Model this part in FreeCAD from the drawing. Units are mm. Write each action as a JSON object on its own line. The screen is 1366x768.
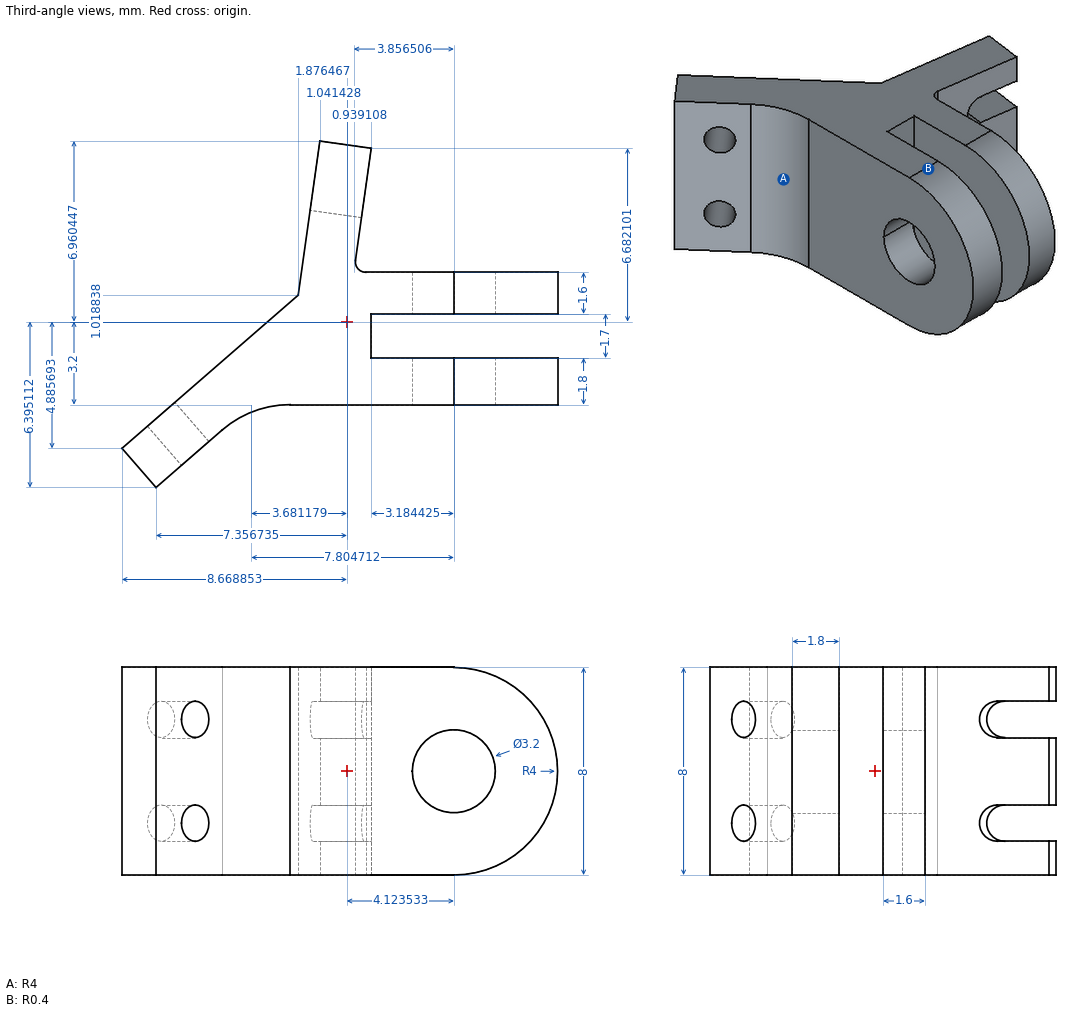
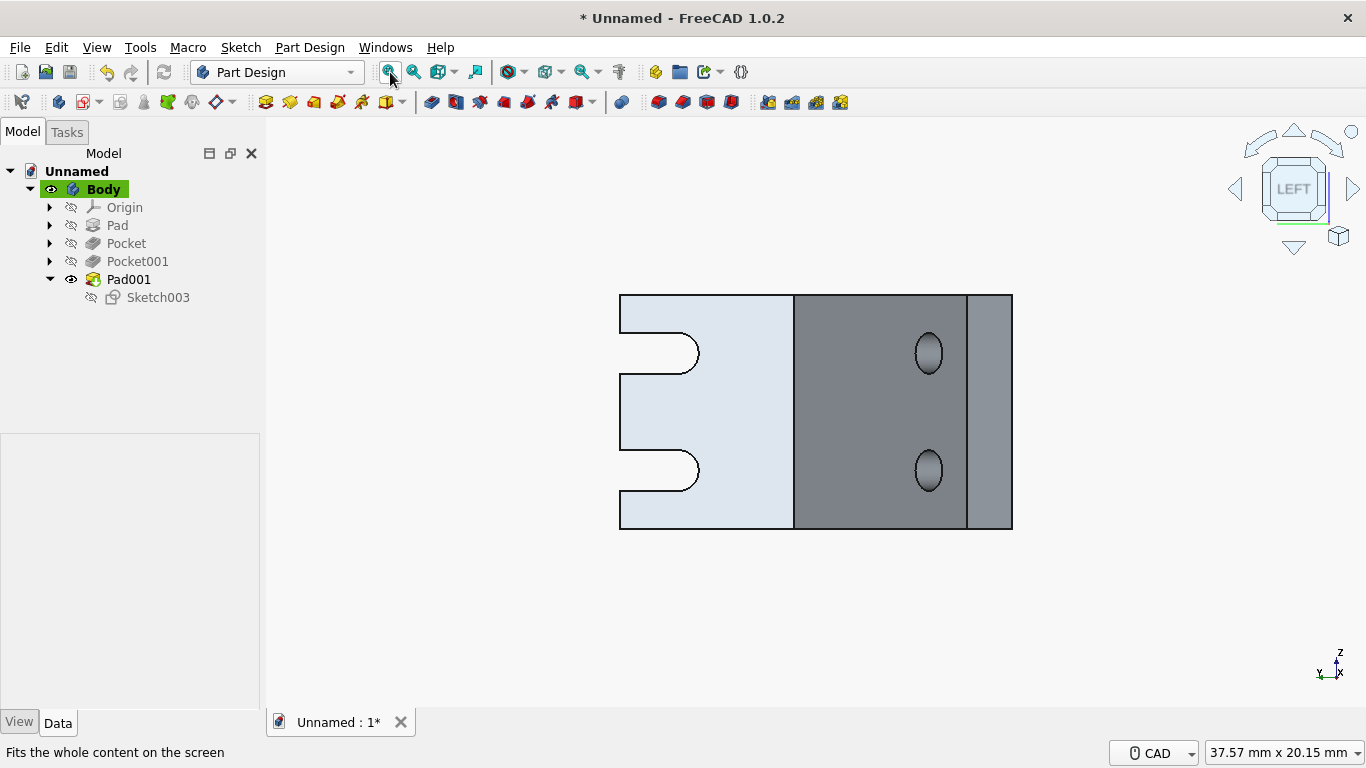
{"action": "key", "text": "v 3"}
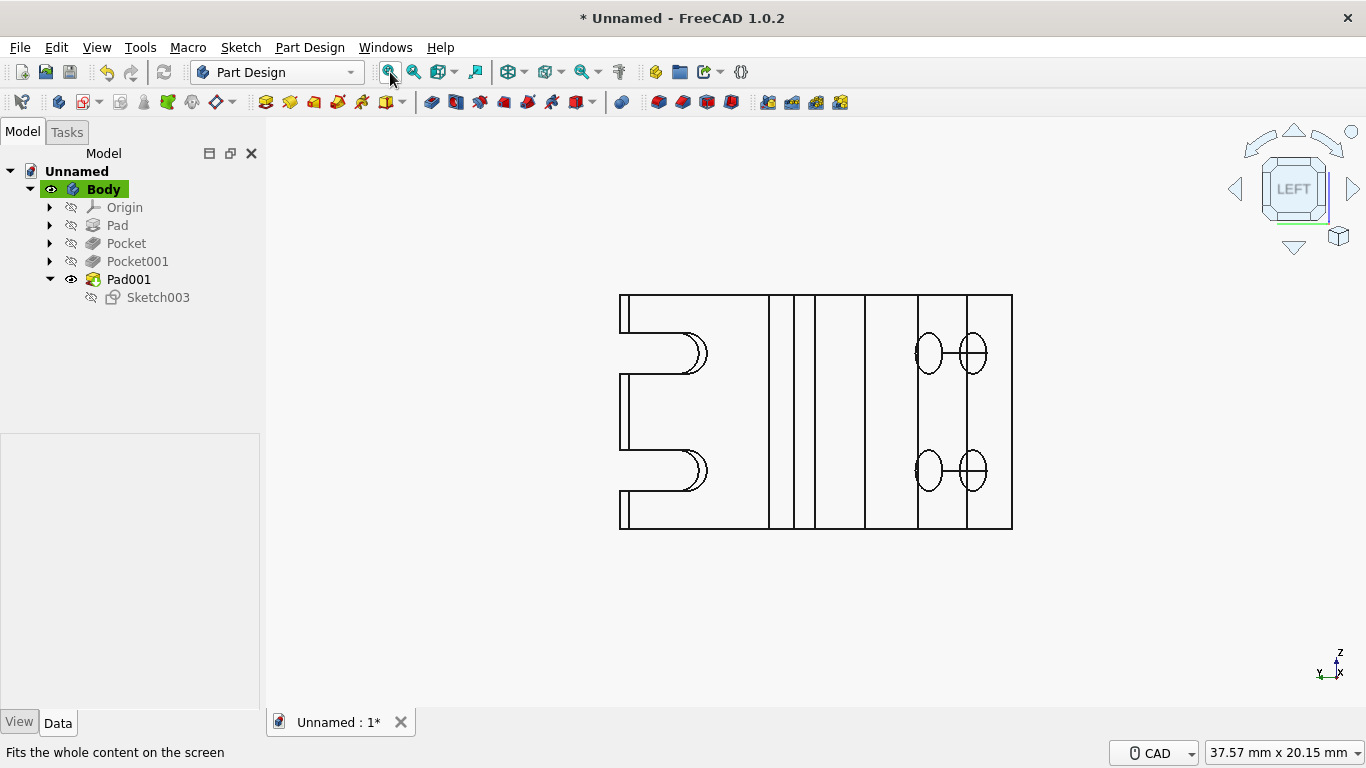
{"action": "key", "text": "0"}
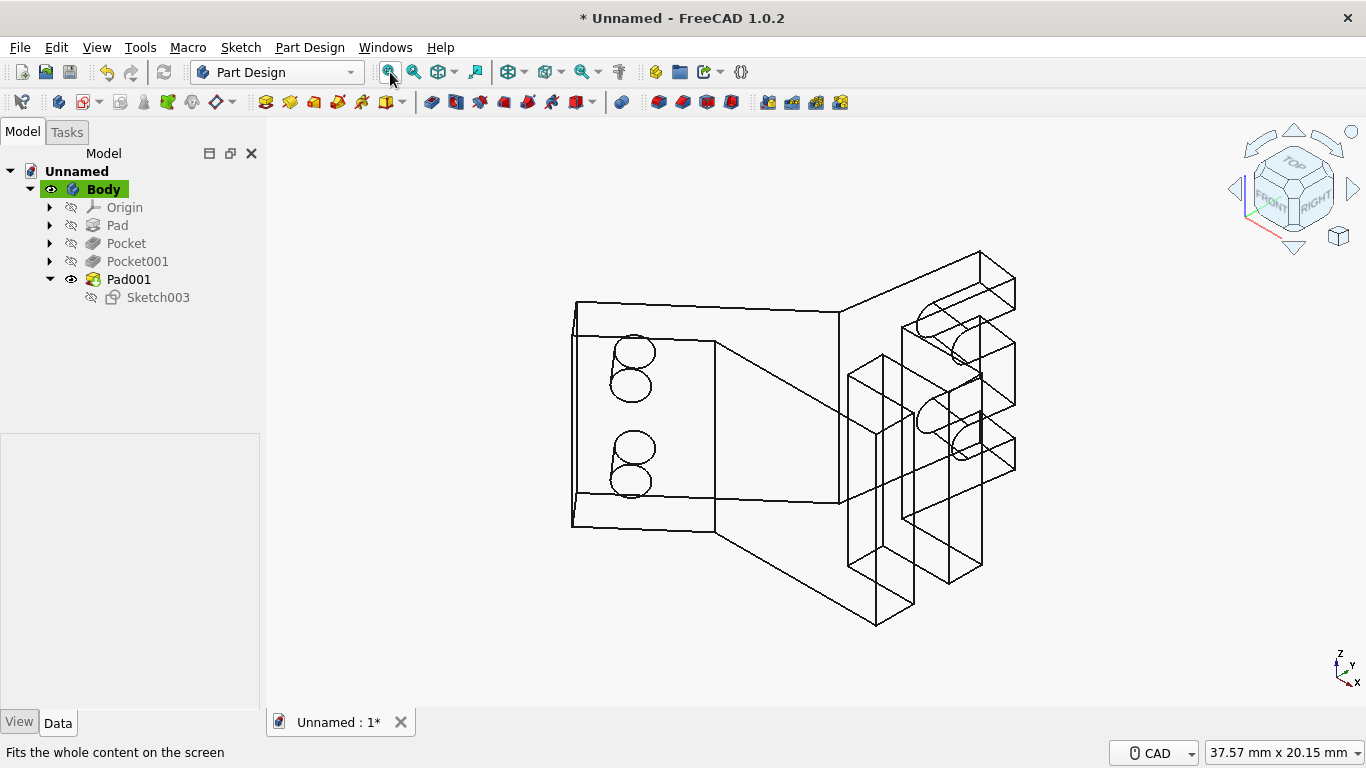
{"action": "left_click", "coordinate": [715, 436]}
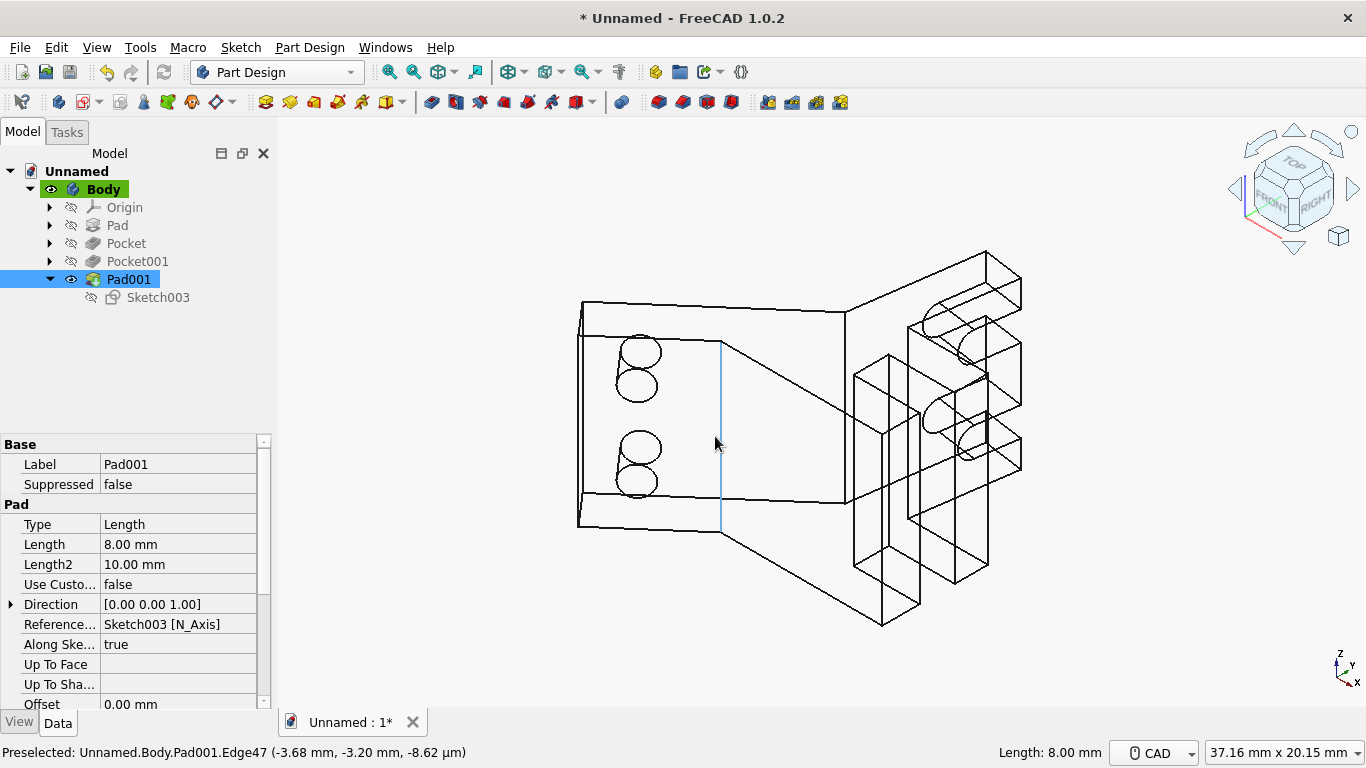
{"action": "key", "text": "v 1"}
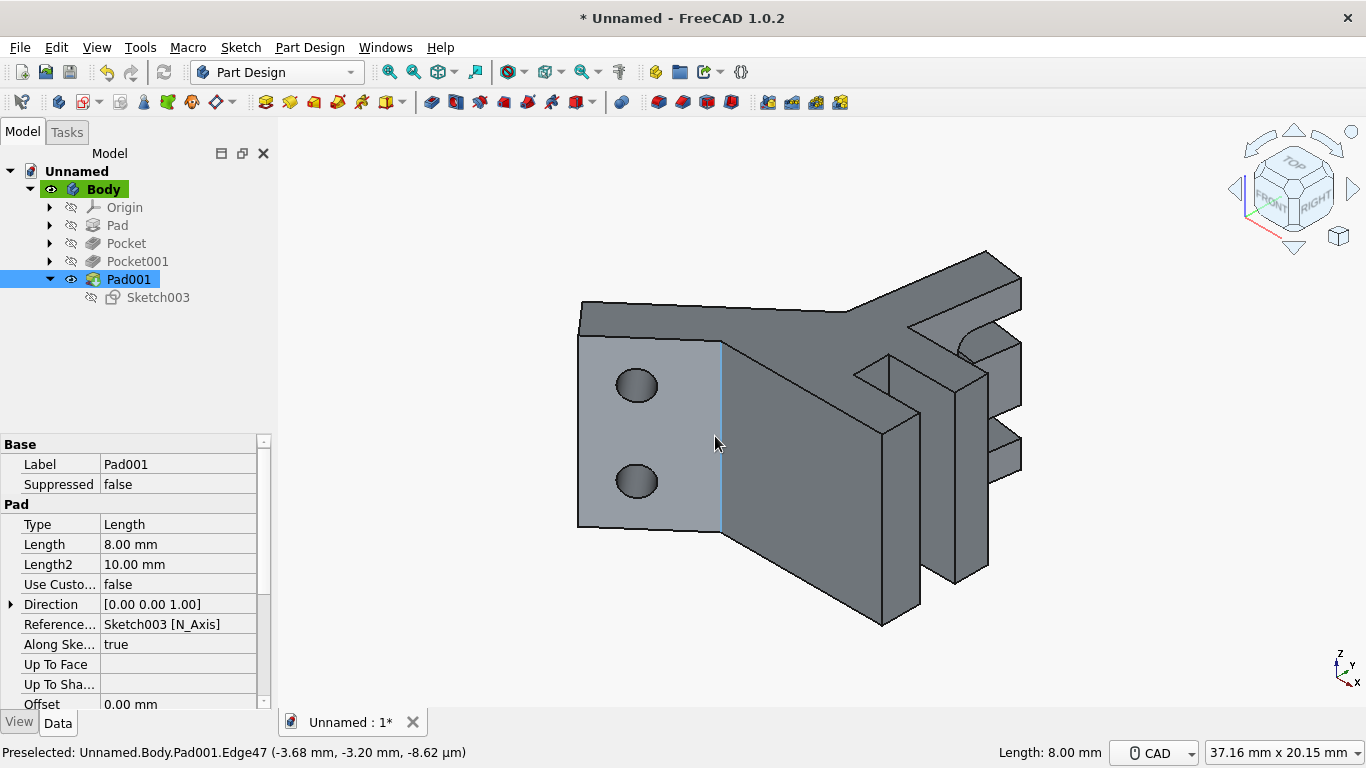
{"action": "left_click", "coordinate": [660, 102]}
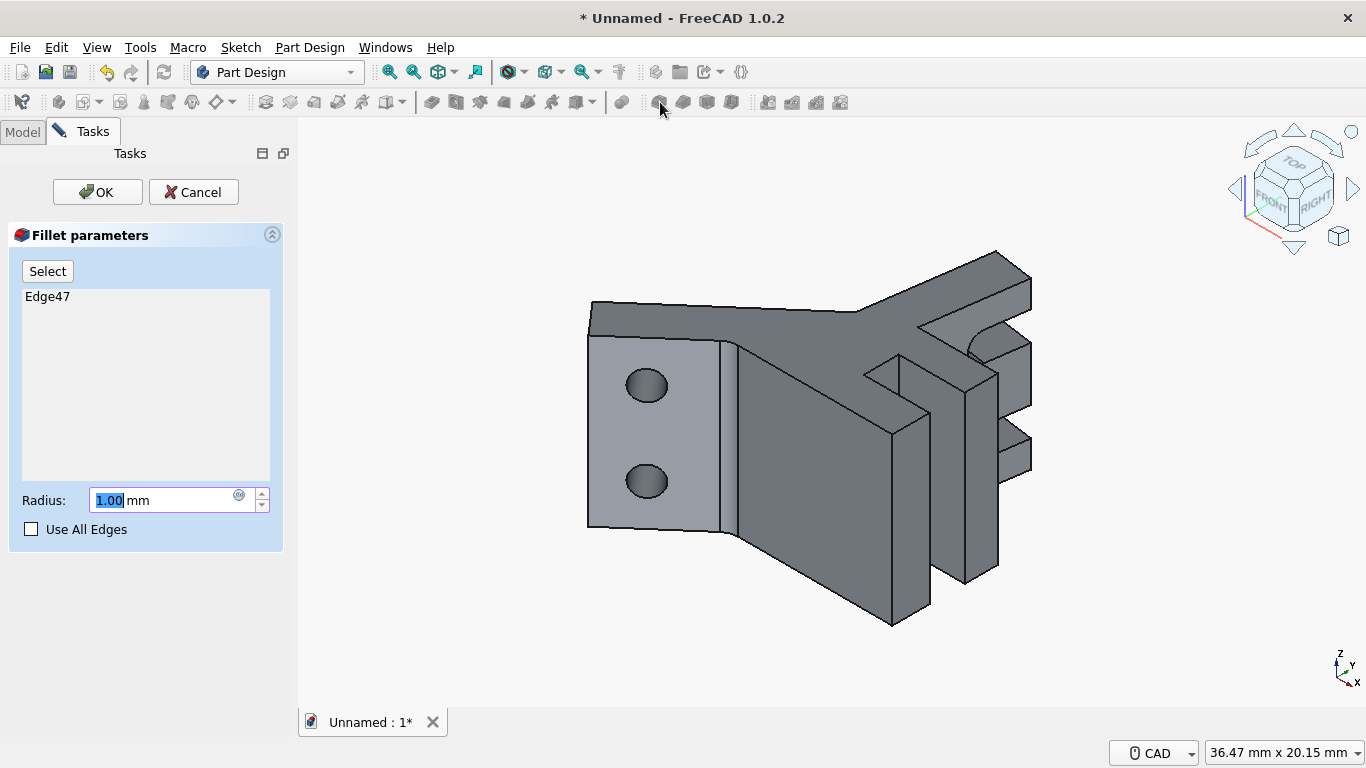
{"action": "type", "text": "4"}
{"action": "key", "text": "Tab"}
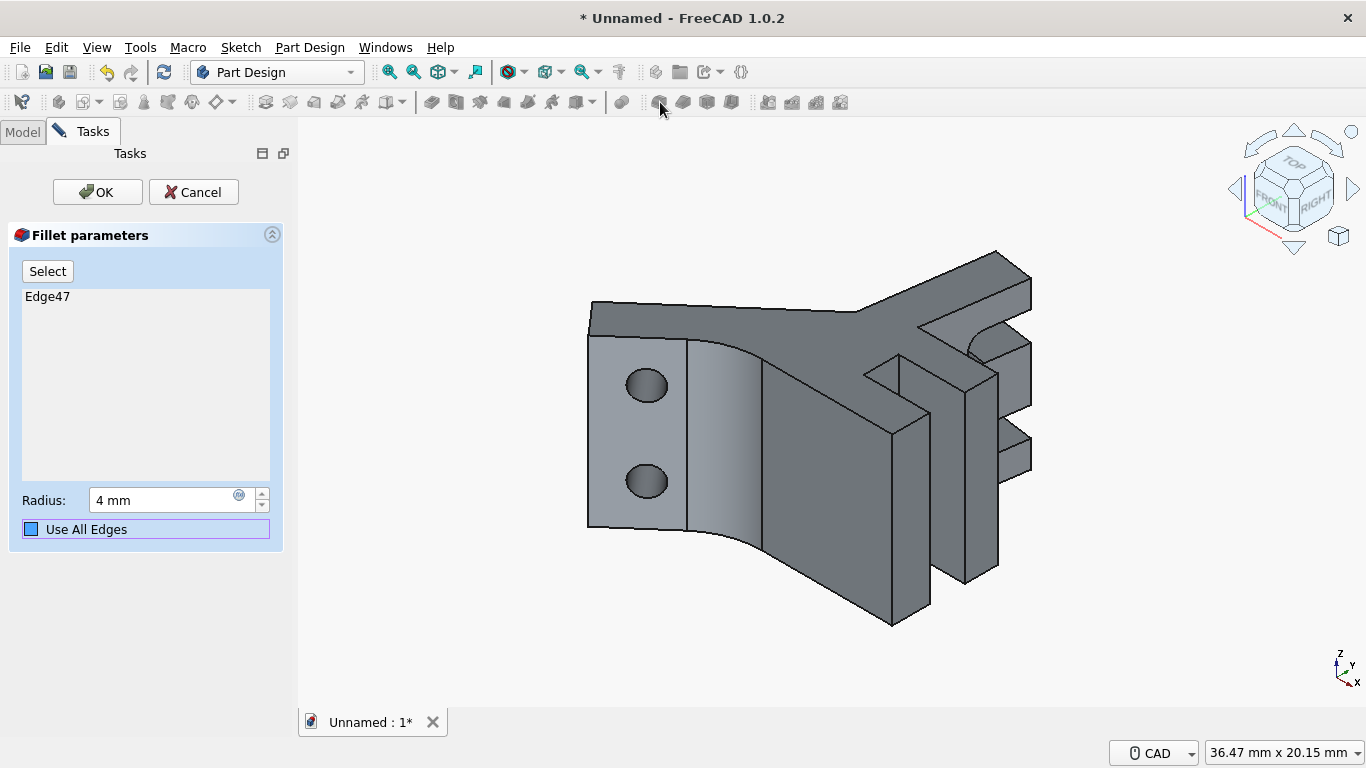
{"action": "left_click", "coordinate": [98, 192]}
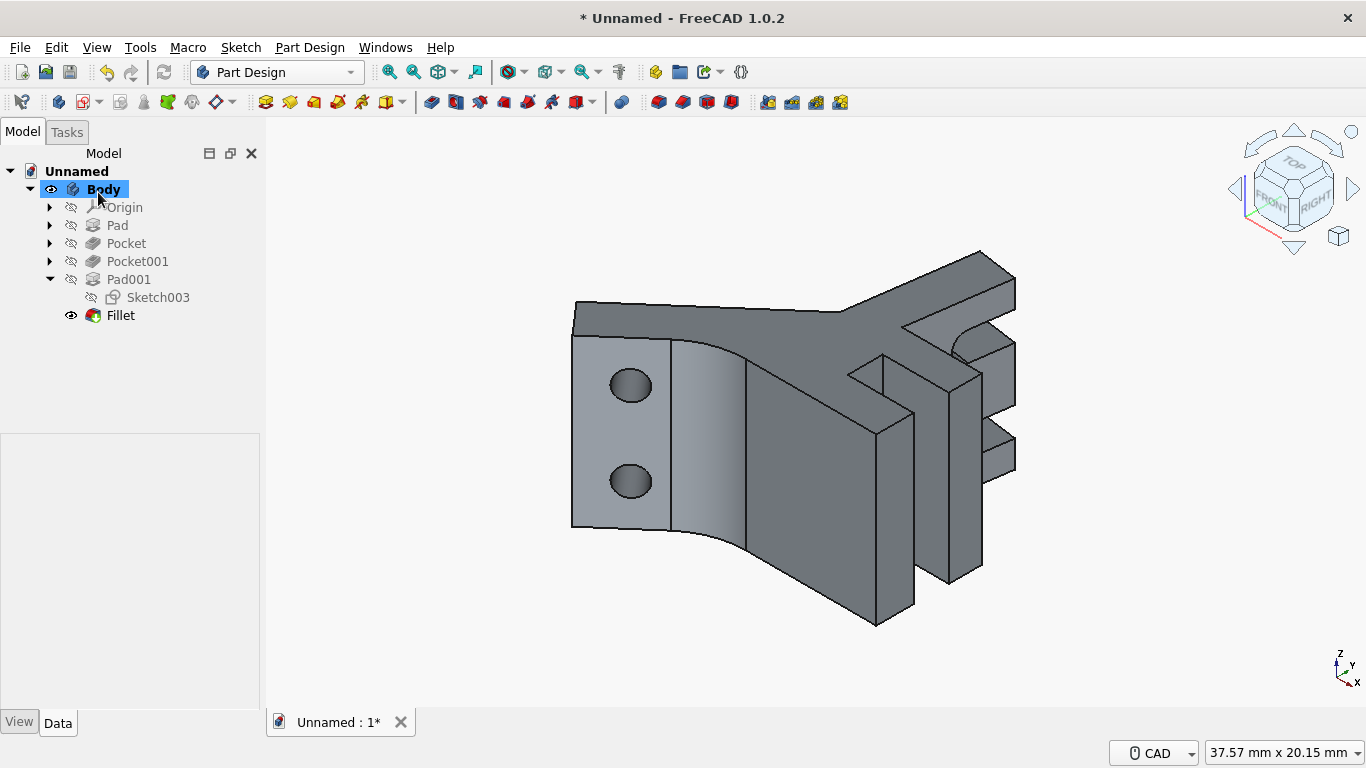
{"action": "key", "text": "2"}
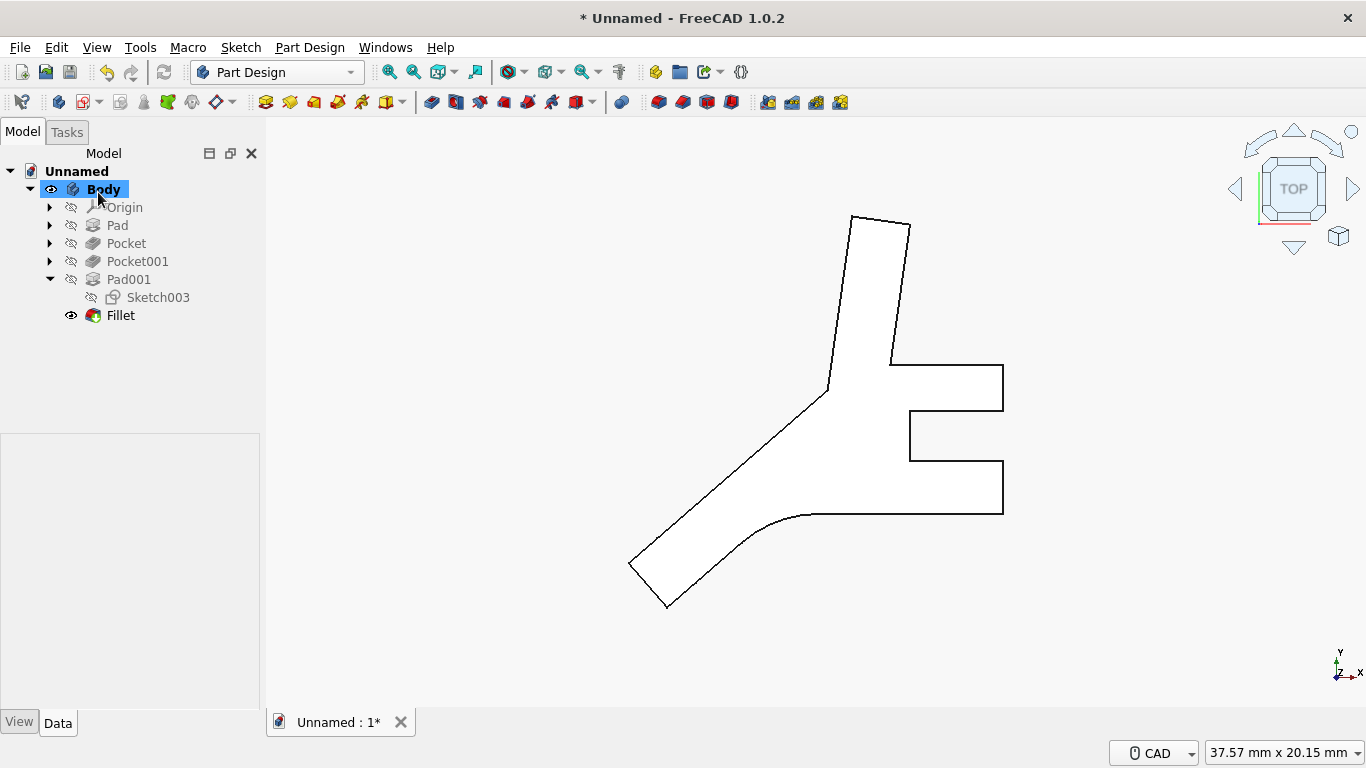
{"action": "key", "text": "0"}